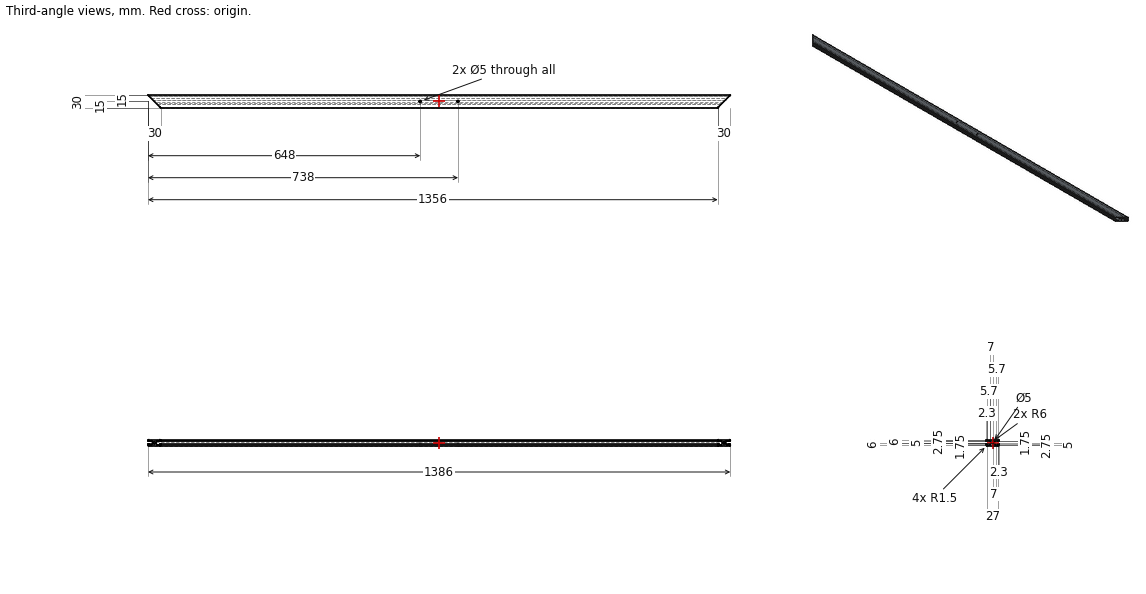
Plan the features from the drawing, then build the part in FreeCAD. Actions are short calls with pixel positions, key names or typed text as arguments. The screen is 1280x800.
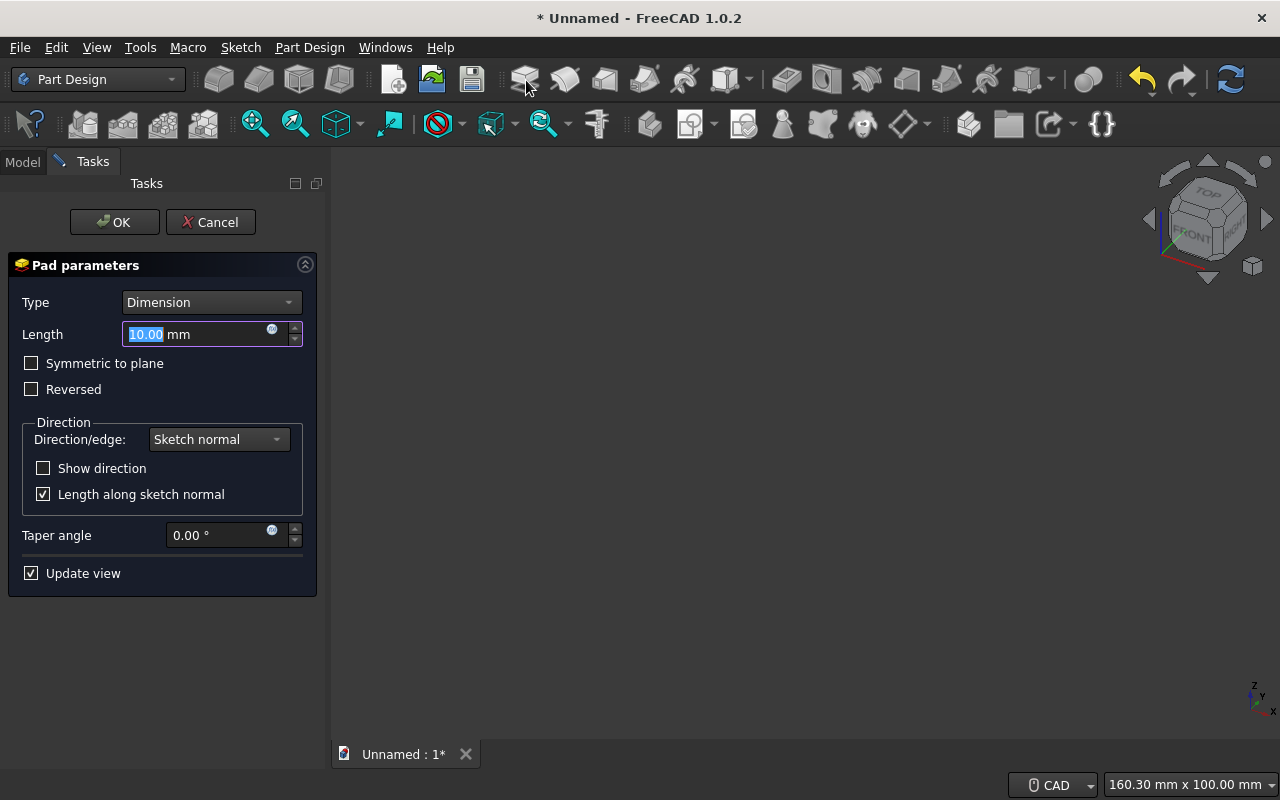
text(1386)
key(Tab)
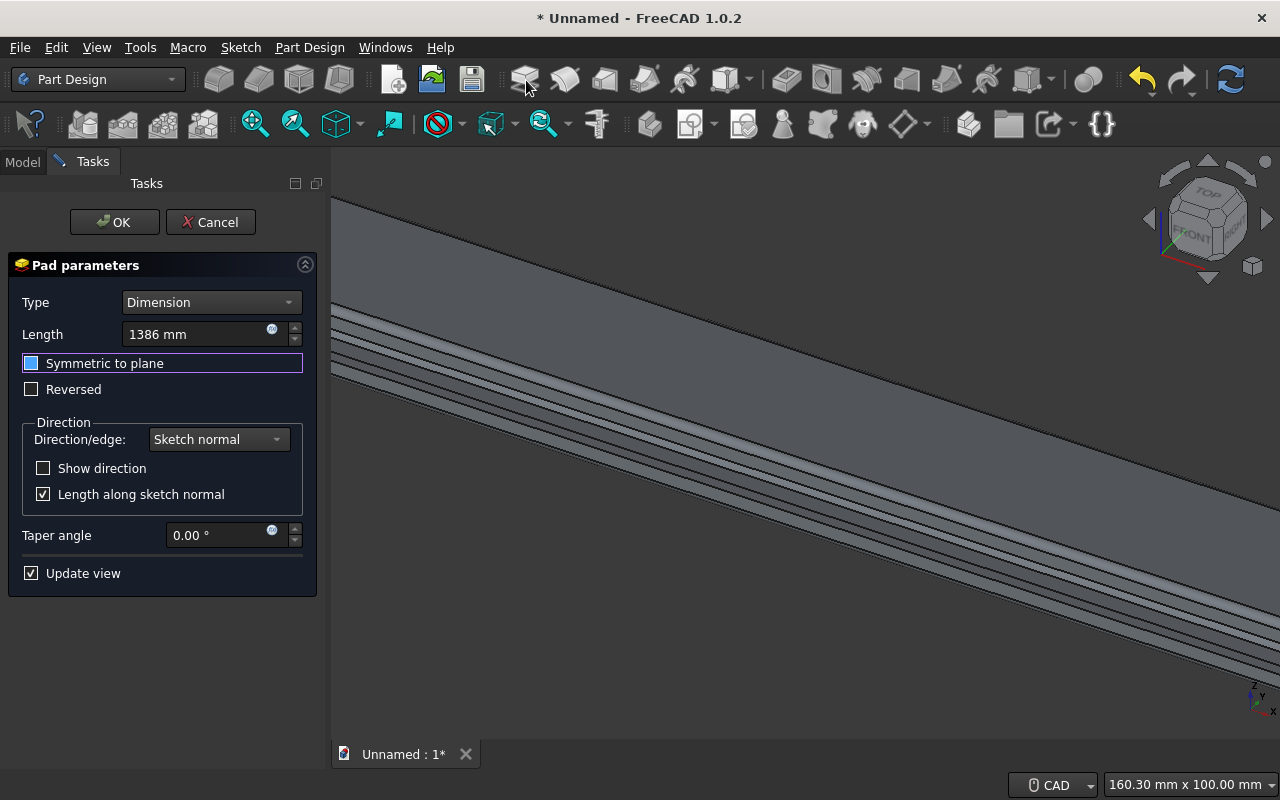
click(115, 222)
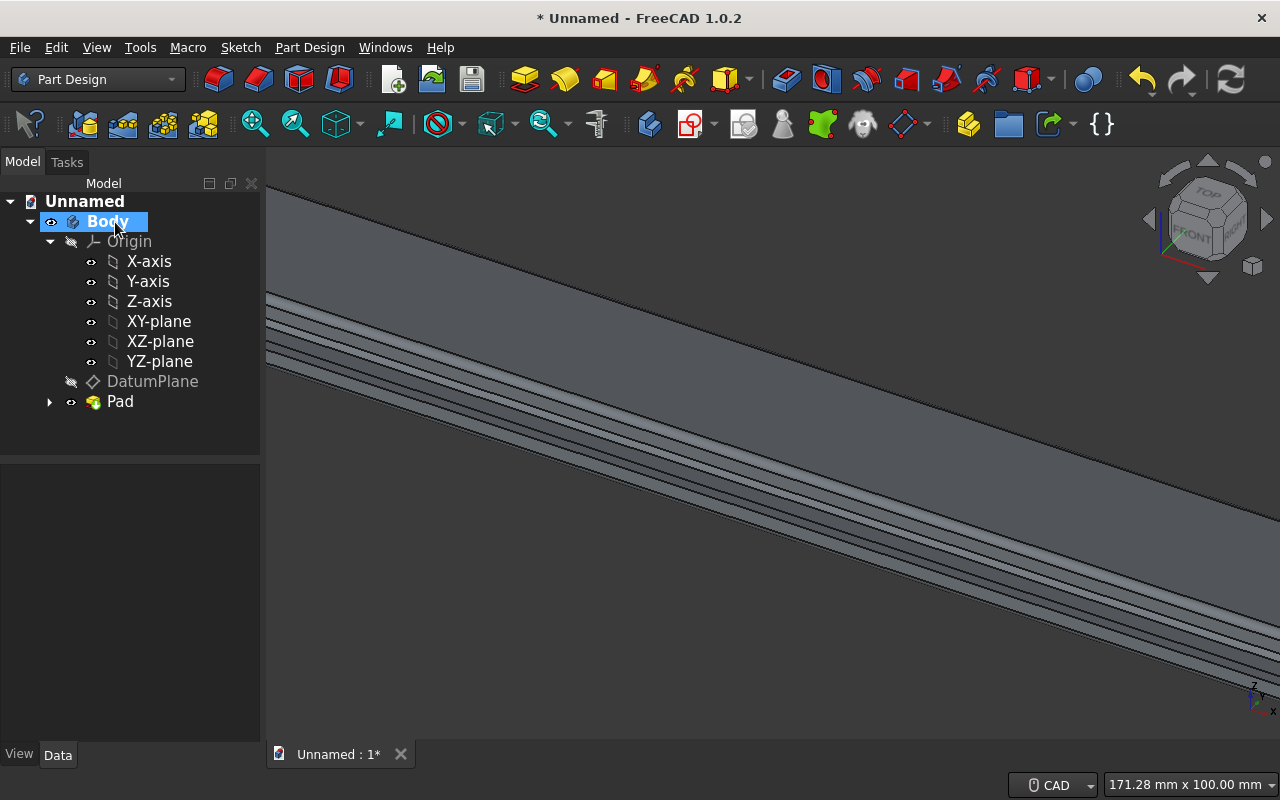
key(v)
key(f)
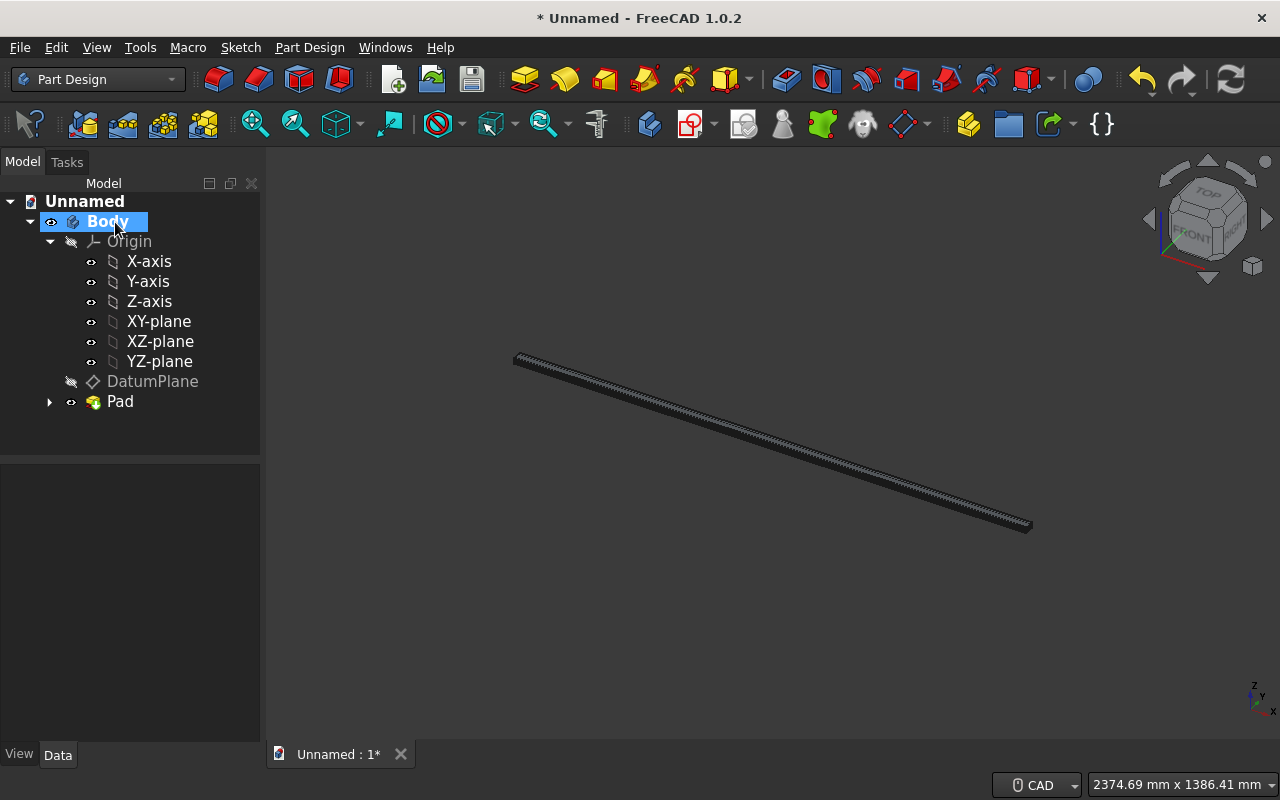
scroll(773, 439, up, 4)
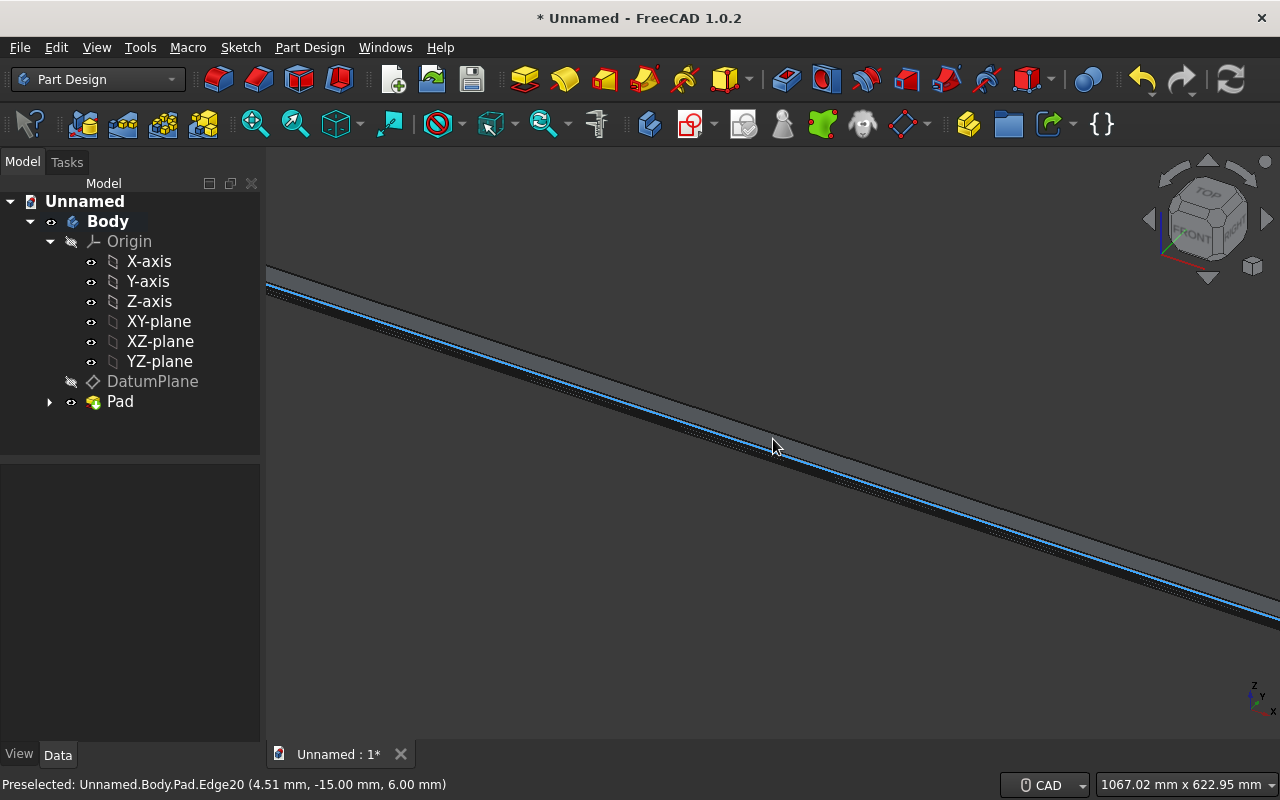
click(256, 124)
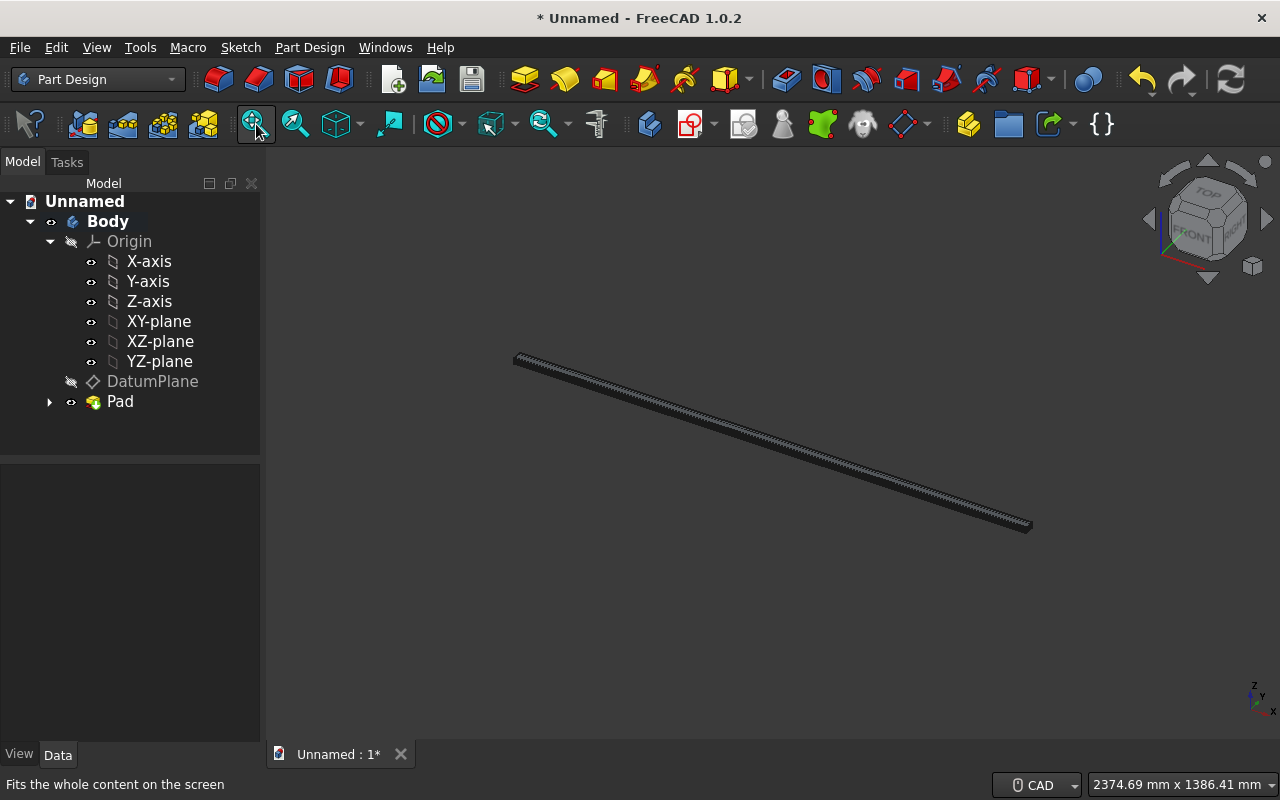
key(0)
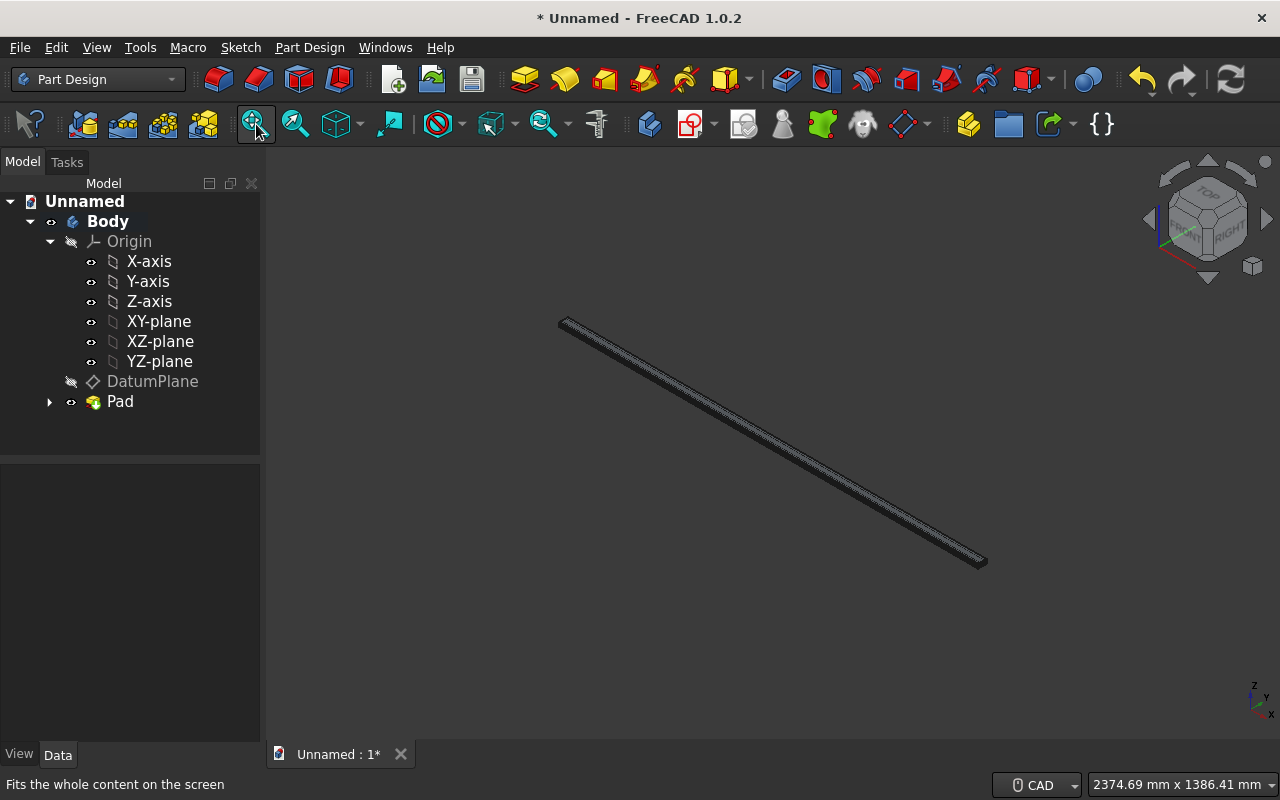
click(256, 124)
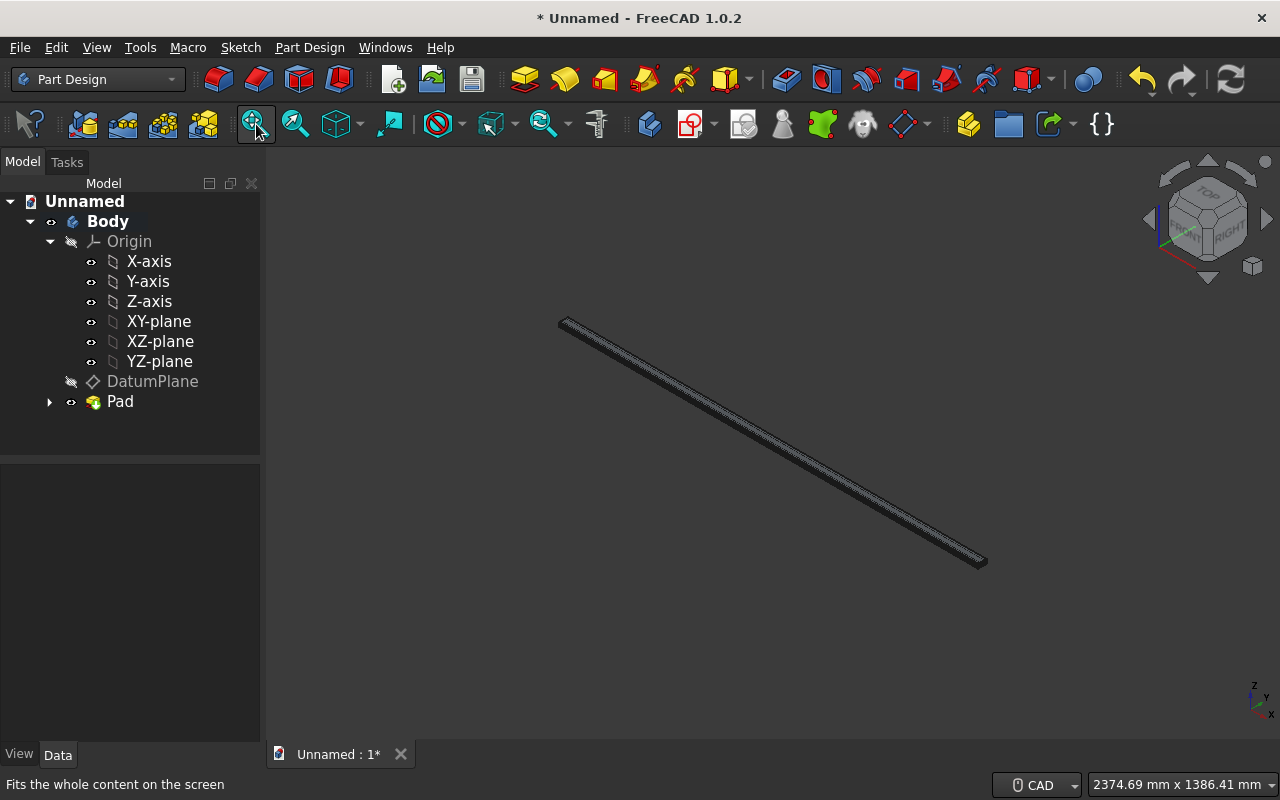
scroll(773, 439, up, 4)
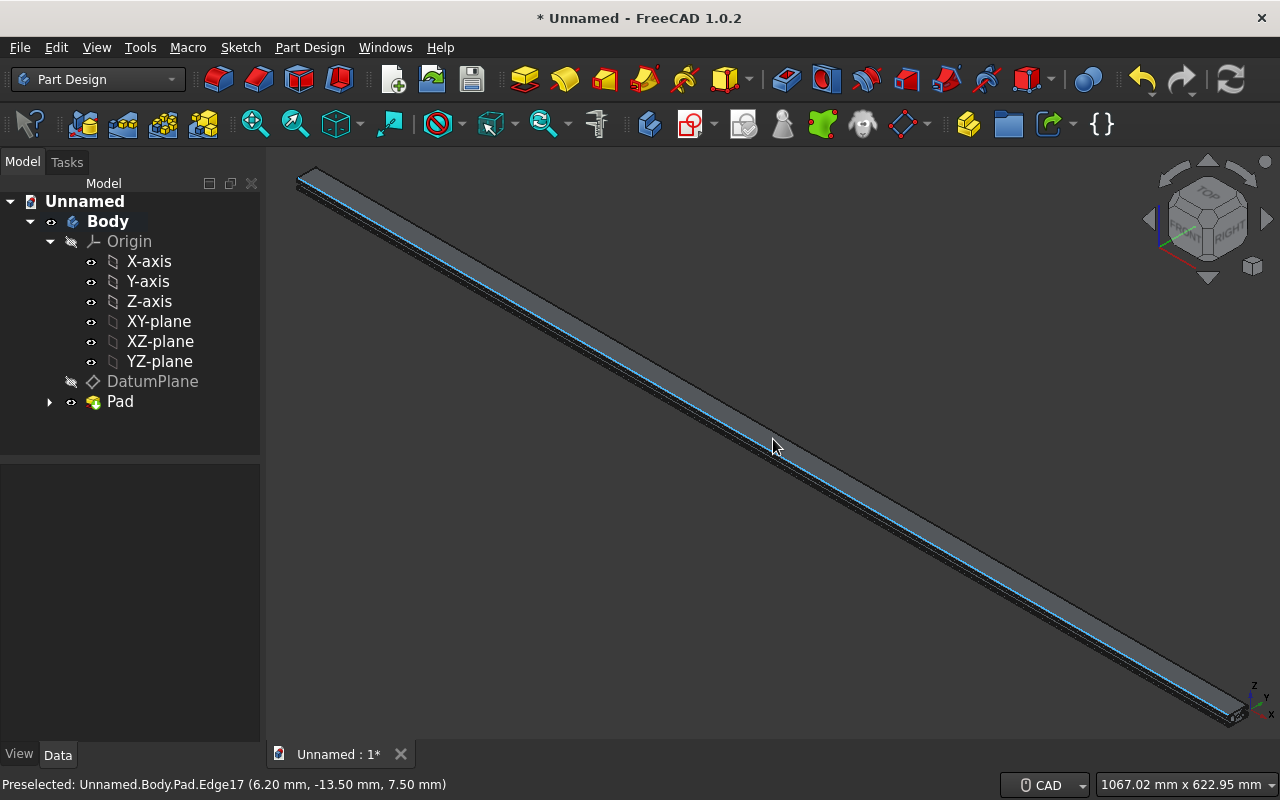
click(772, 440)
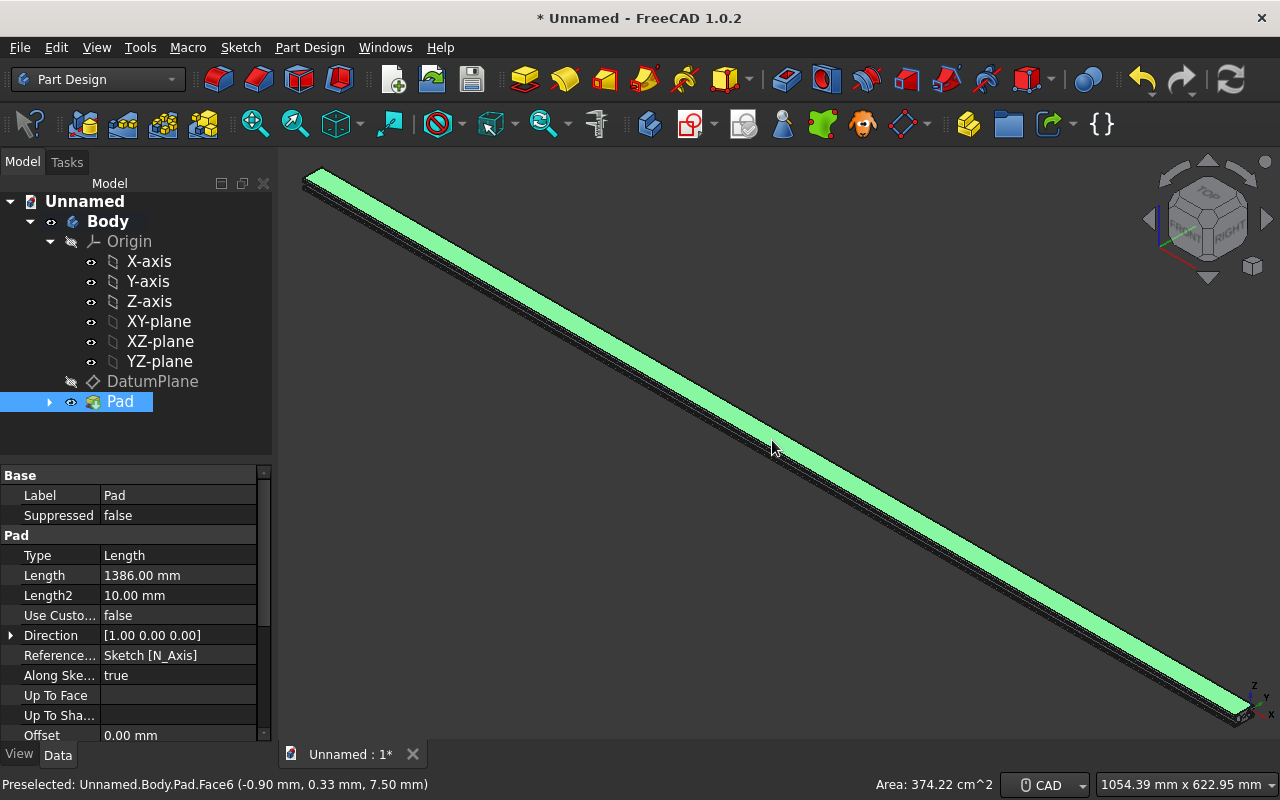
click(690, 124)